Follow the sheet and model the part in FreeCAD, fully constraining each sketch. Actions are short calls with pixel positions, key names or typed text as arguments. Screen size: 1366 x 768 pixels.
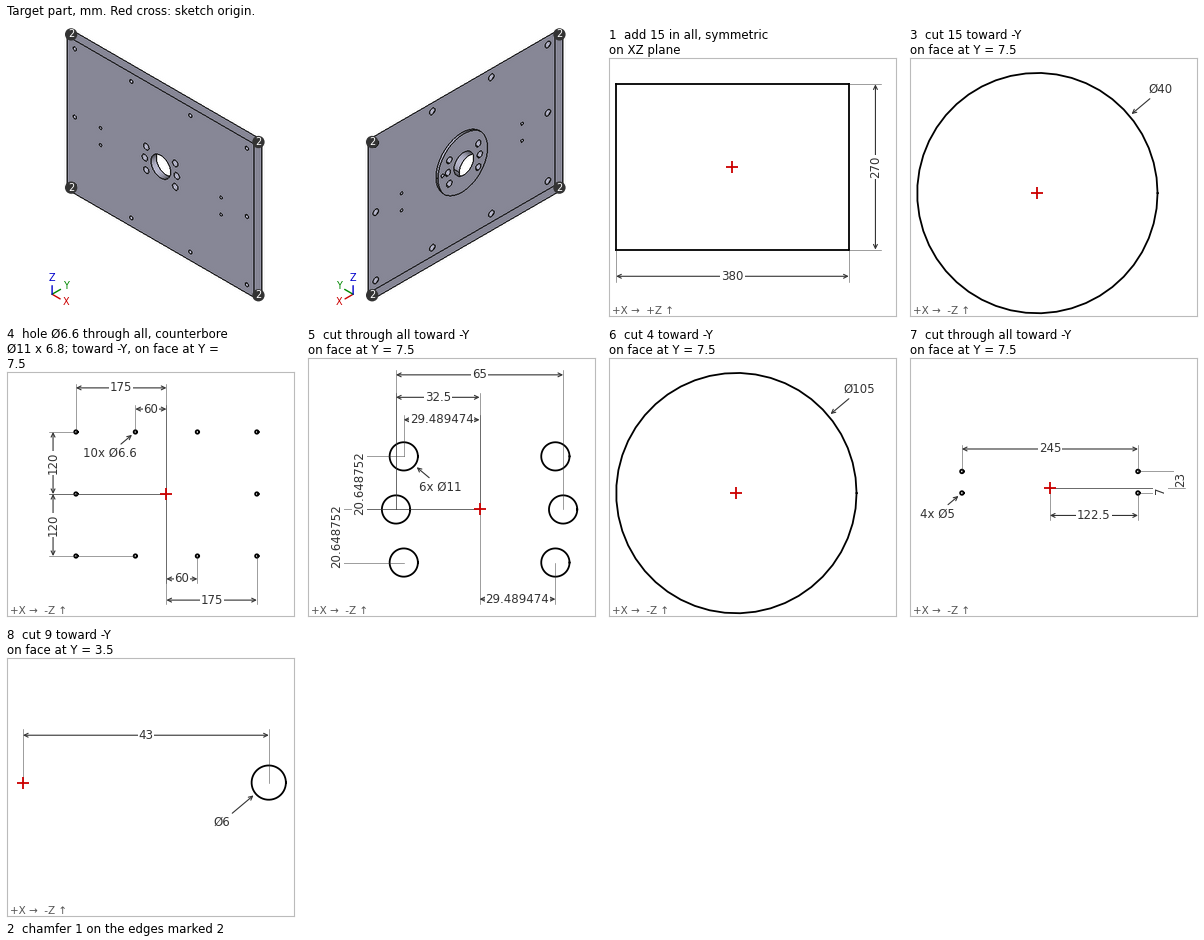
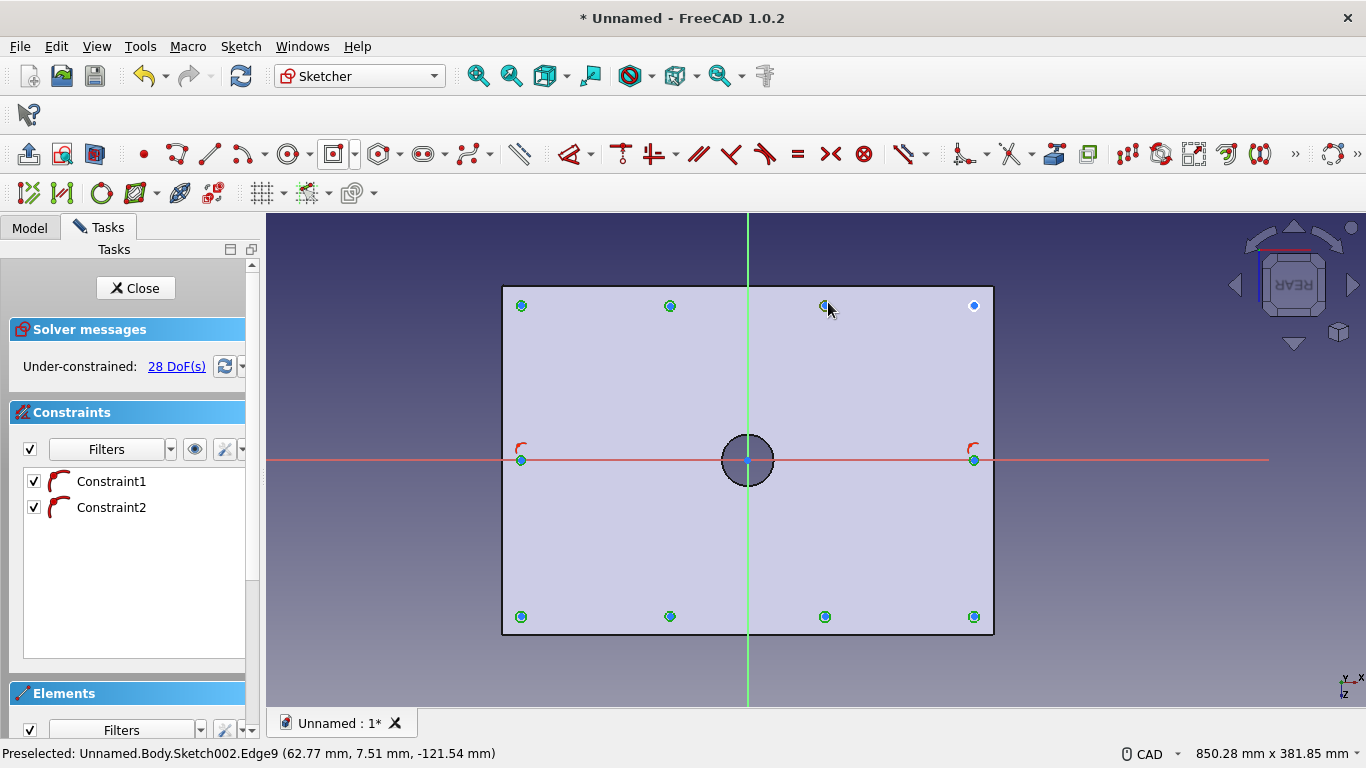
scroll(977, 303, up, 6)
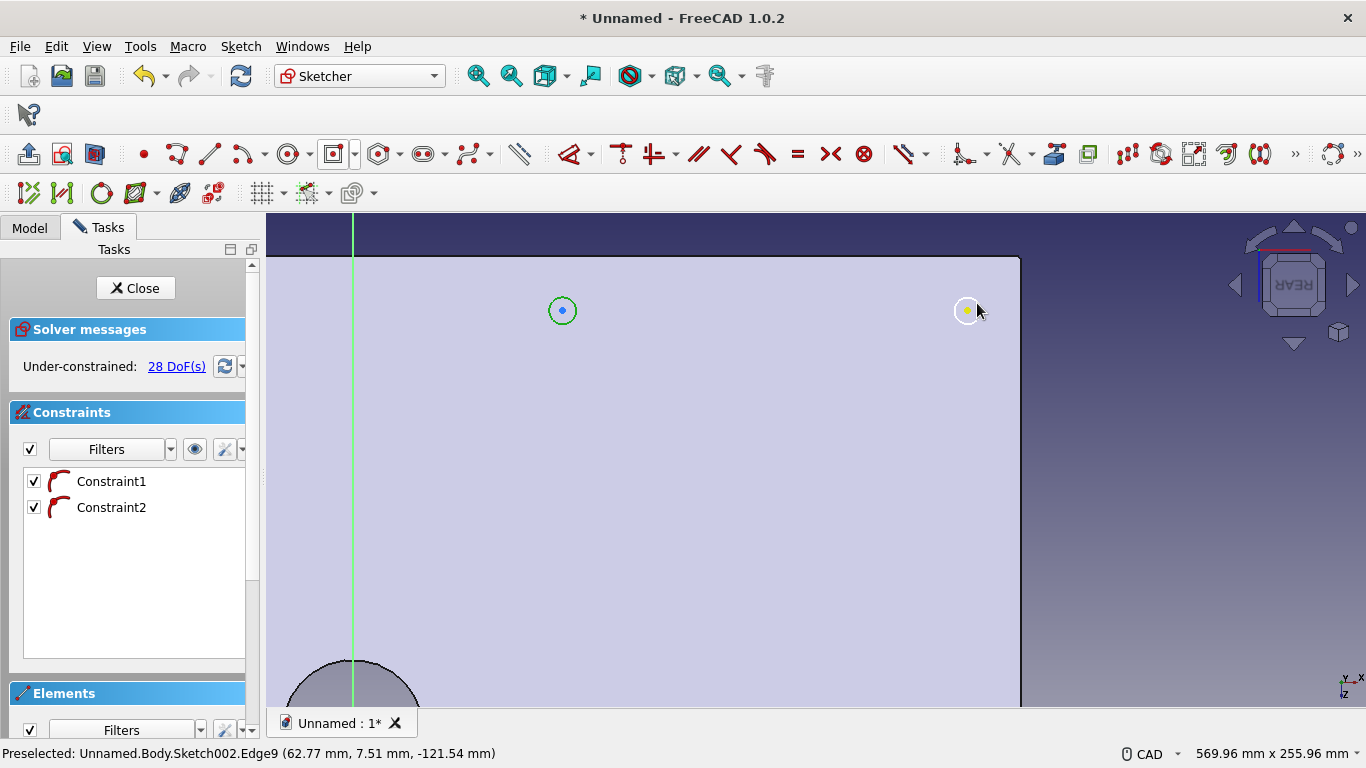
click(977, 301)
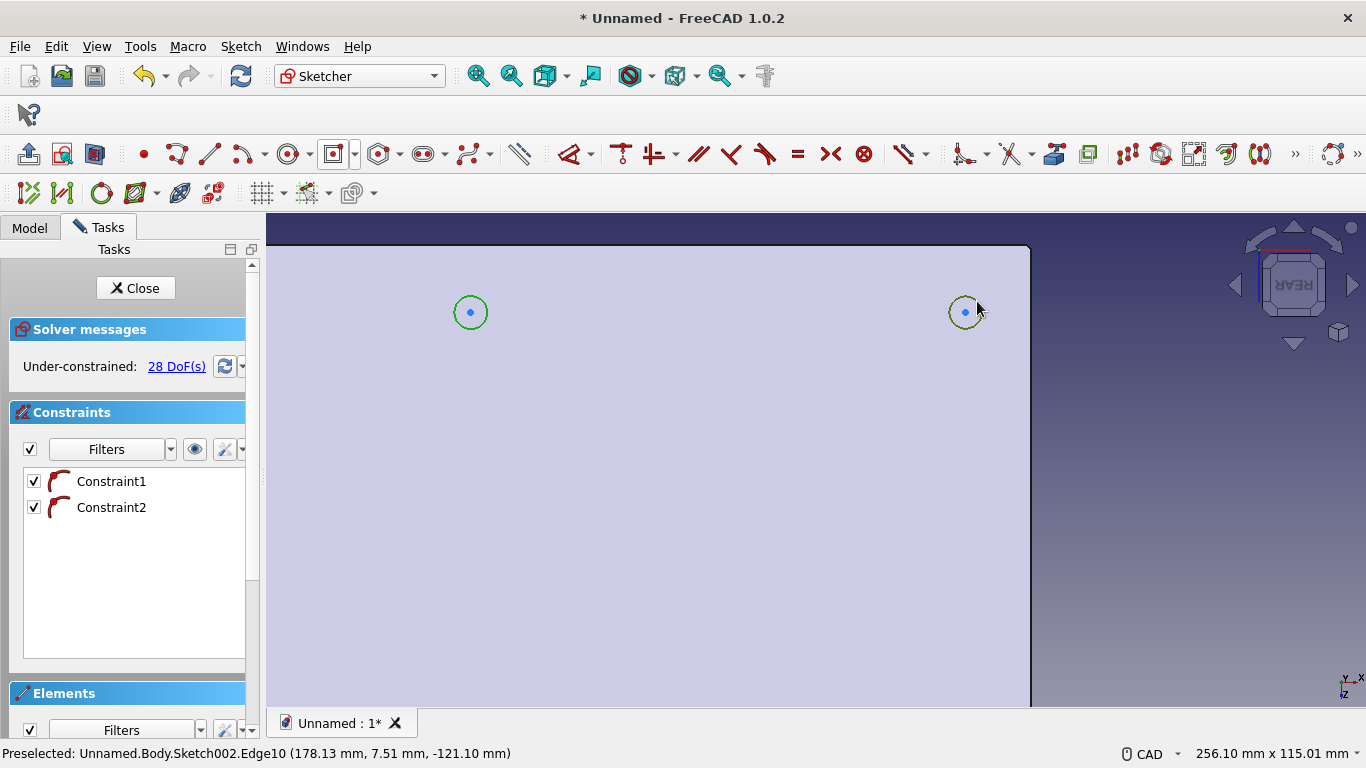
click(798, 154)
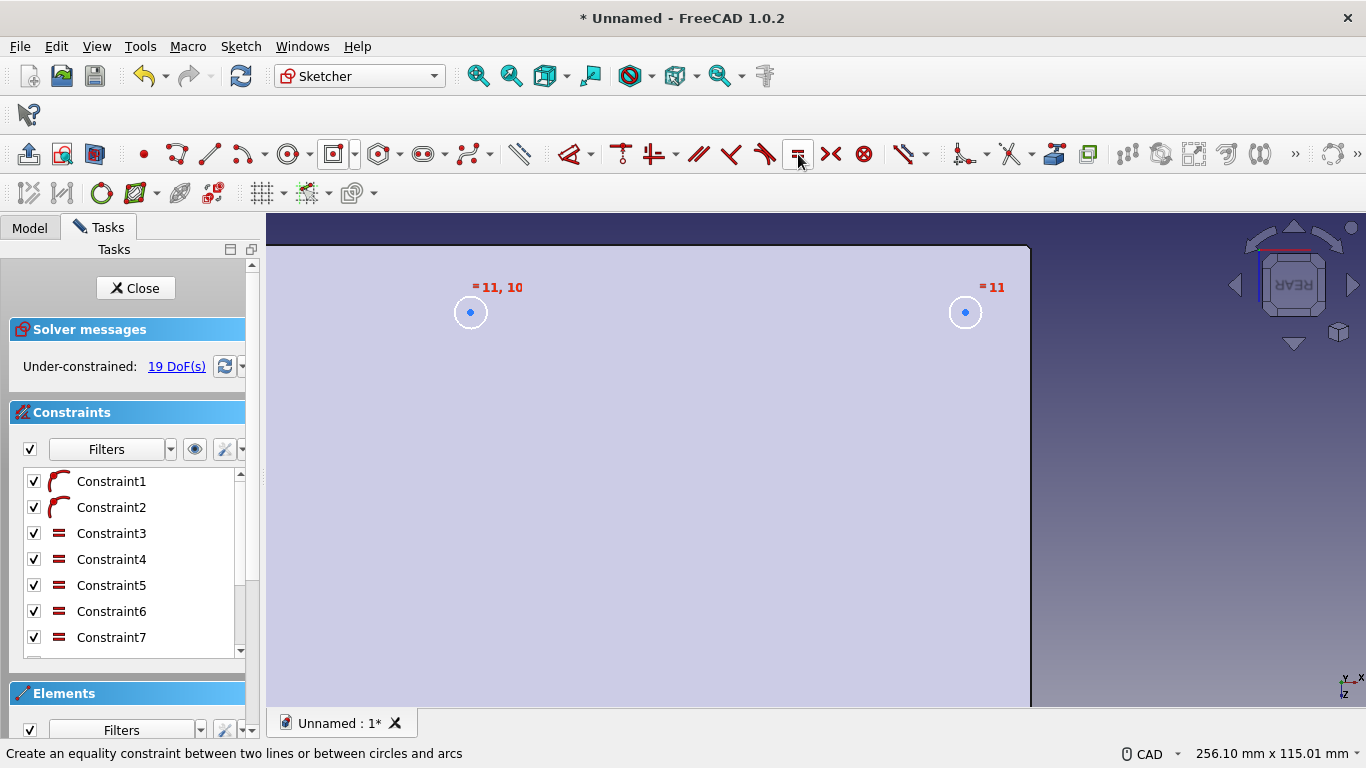
scroll(977, 303, down, 6)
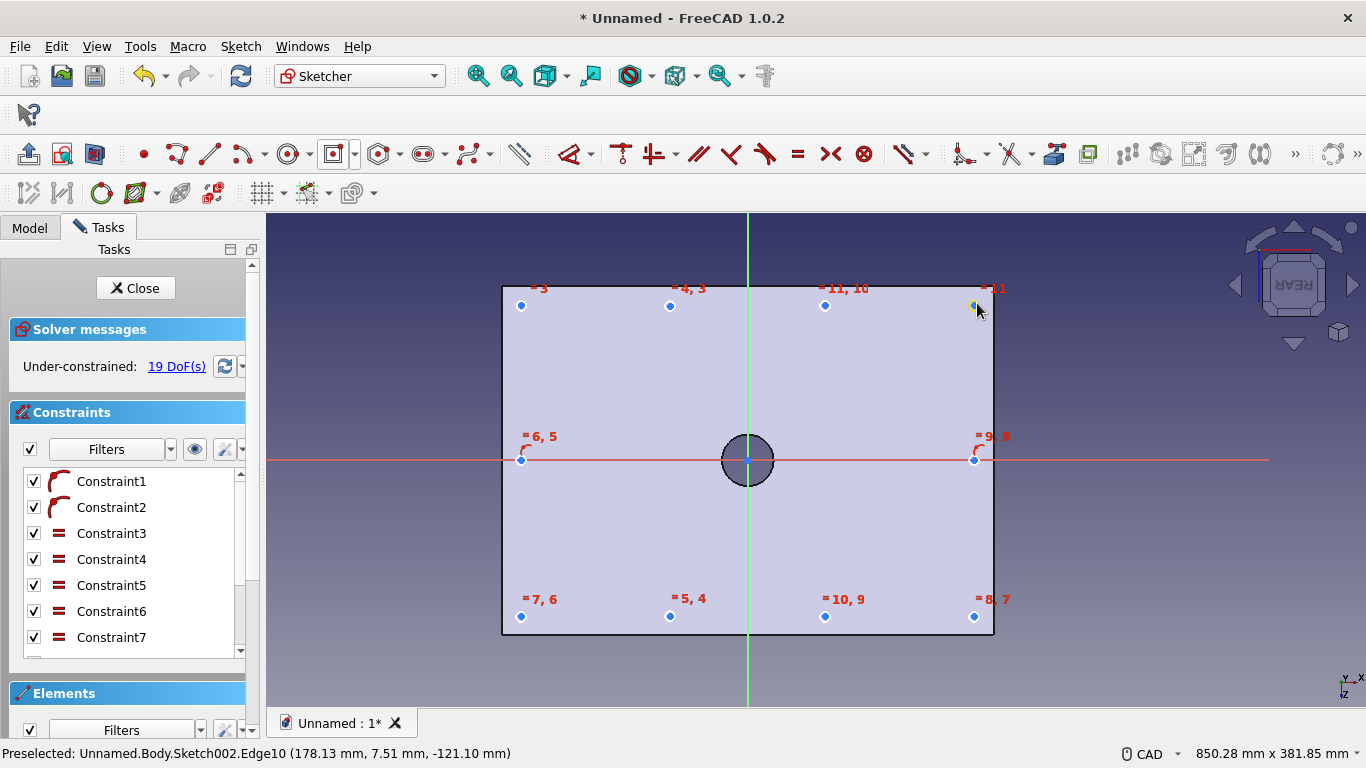
click(521, 306)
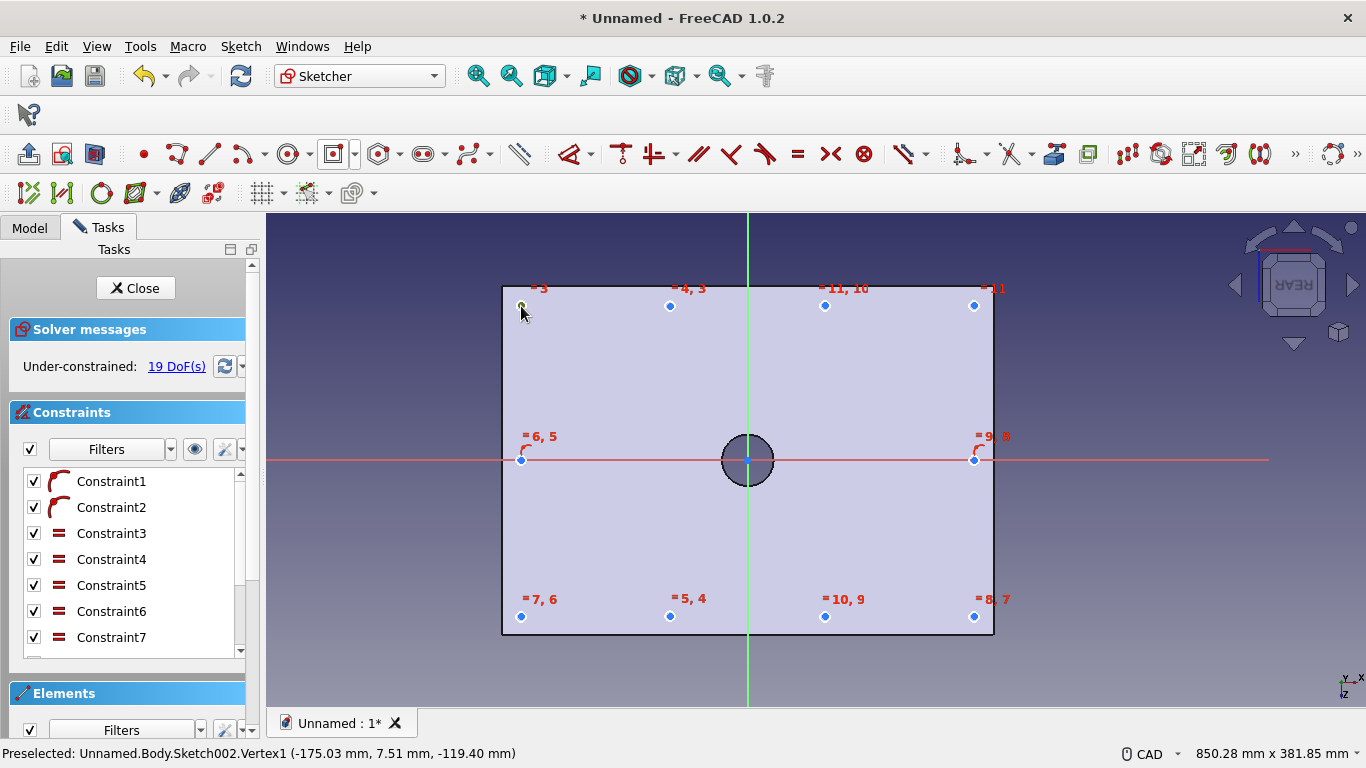
click(670, 306)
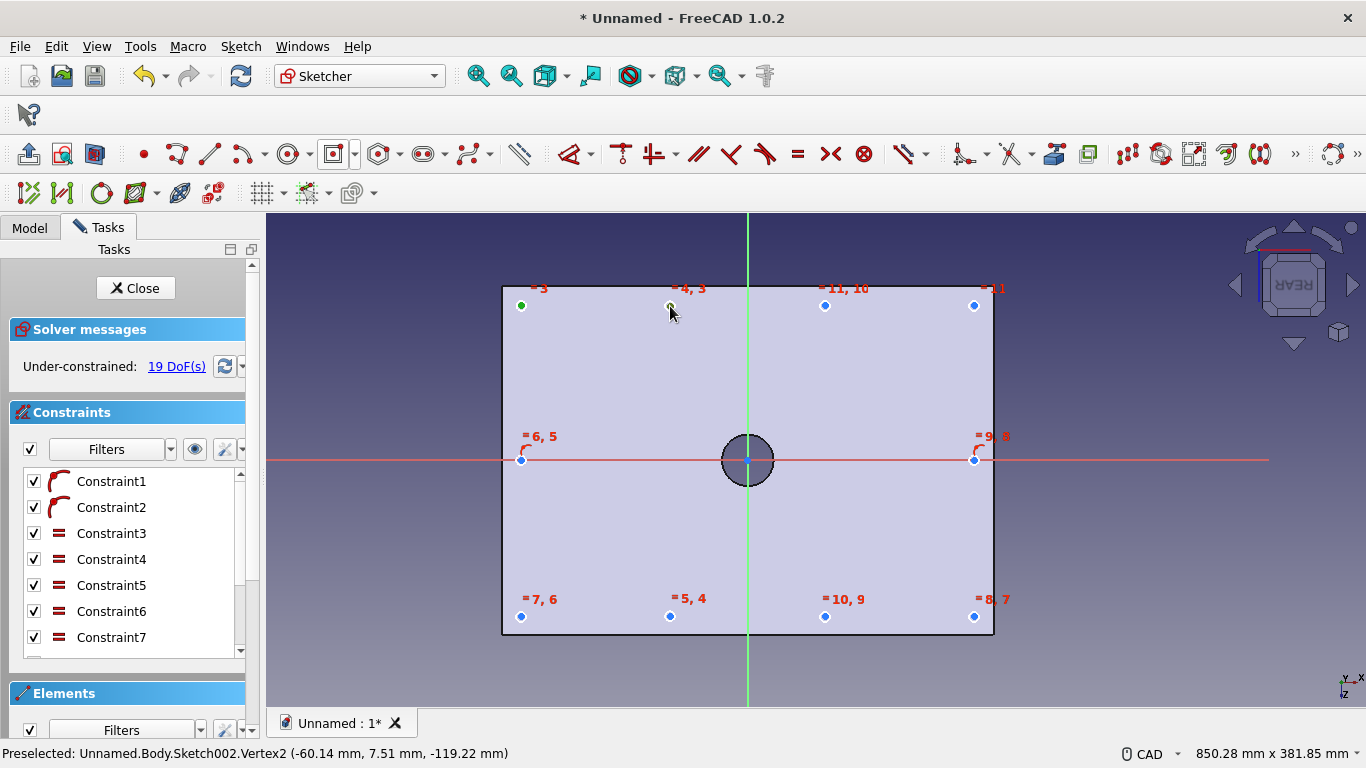
click(676, 154)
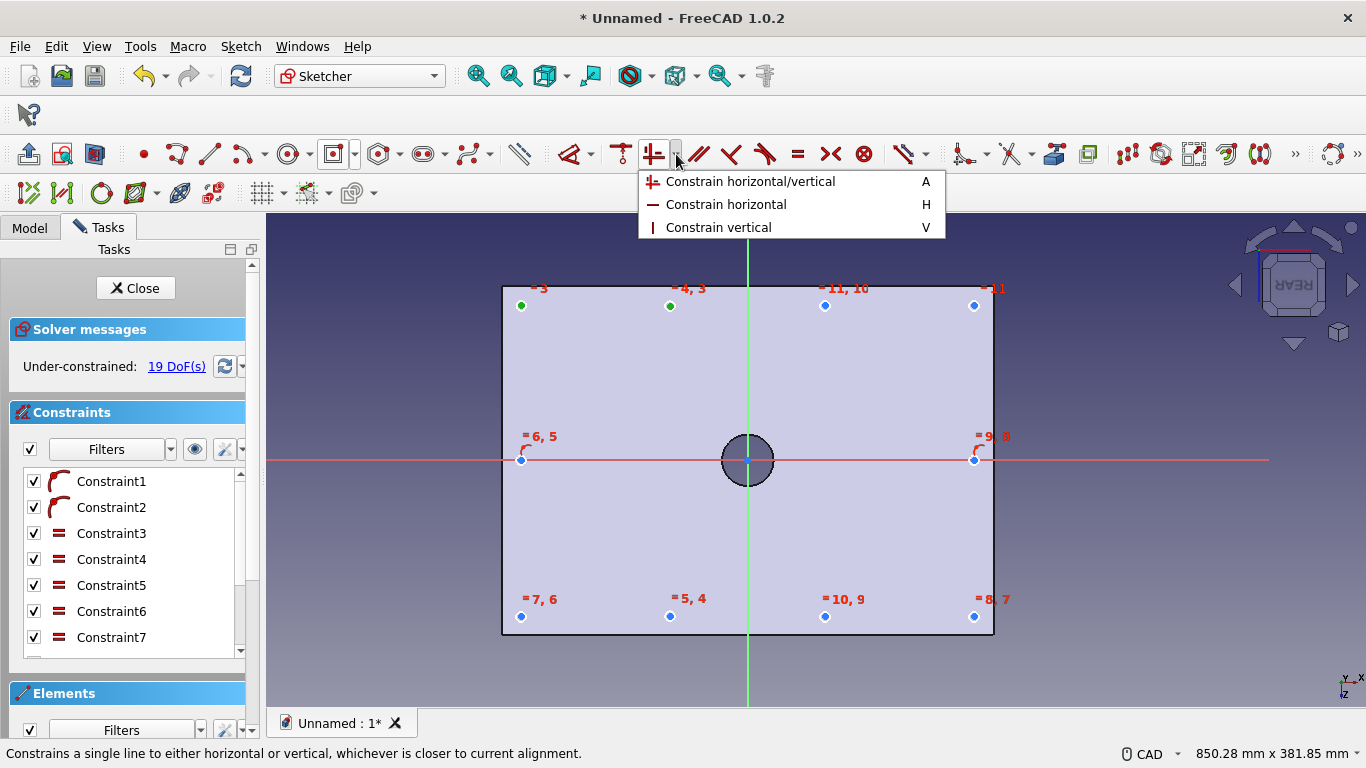
click(792, 204)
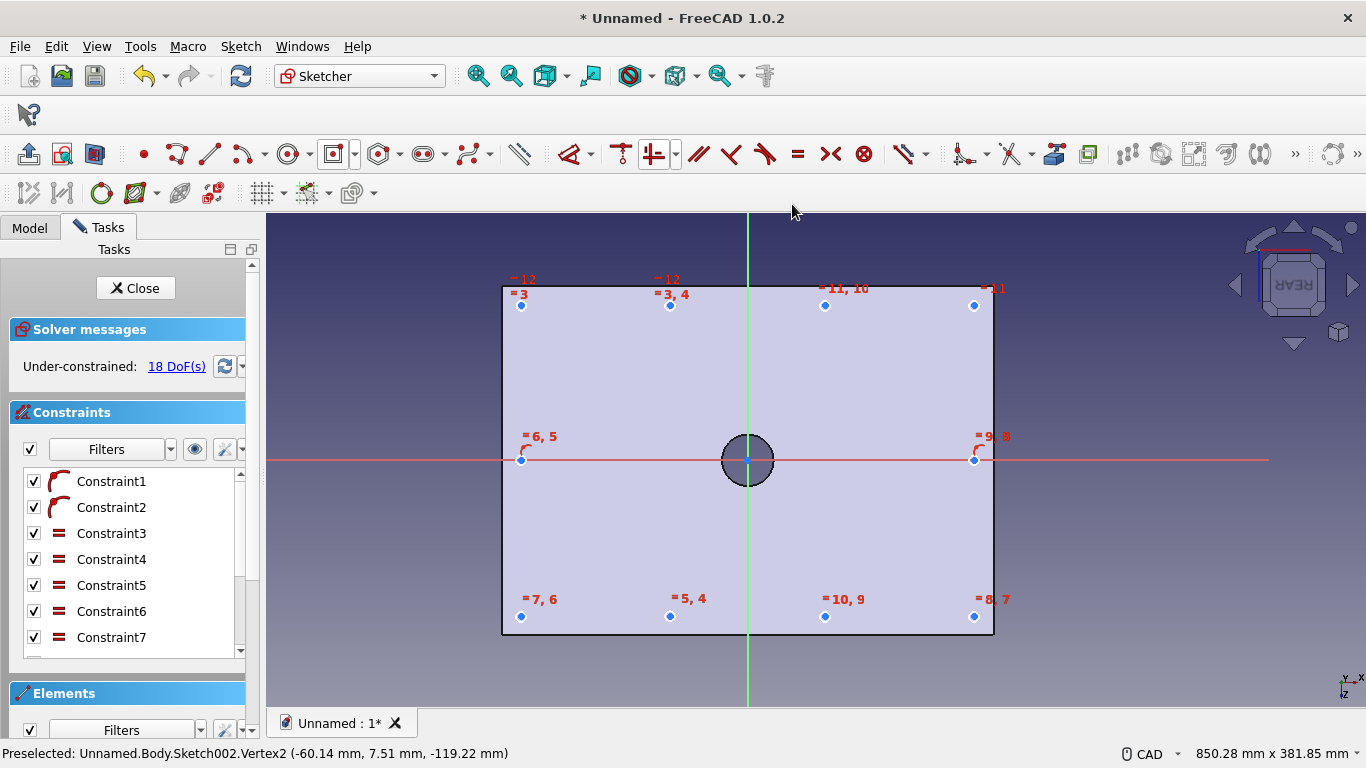
click(670, 306)